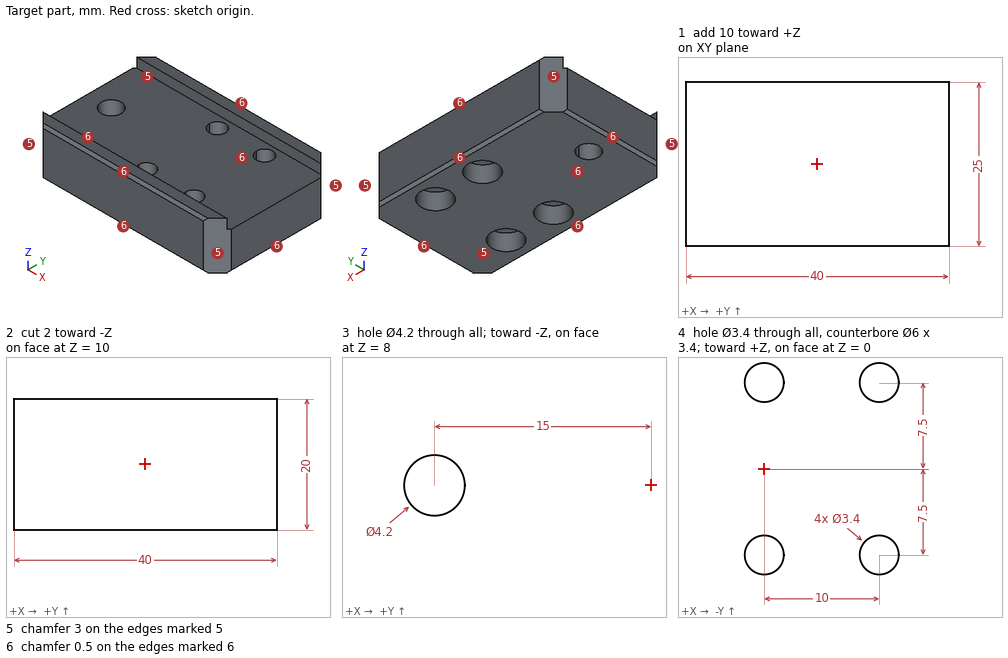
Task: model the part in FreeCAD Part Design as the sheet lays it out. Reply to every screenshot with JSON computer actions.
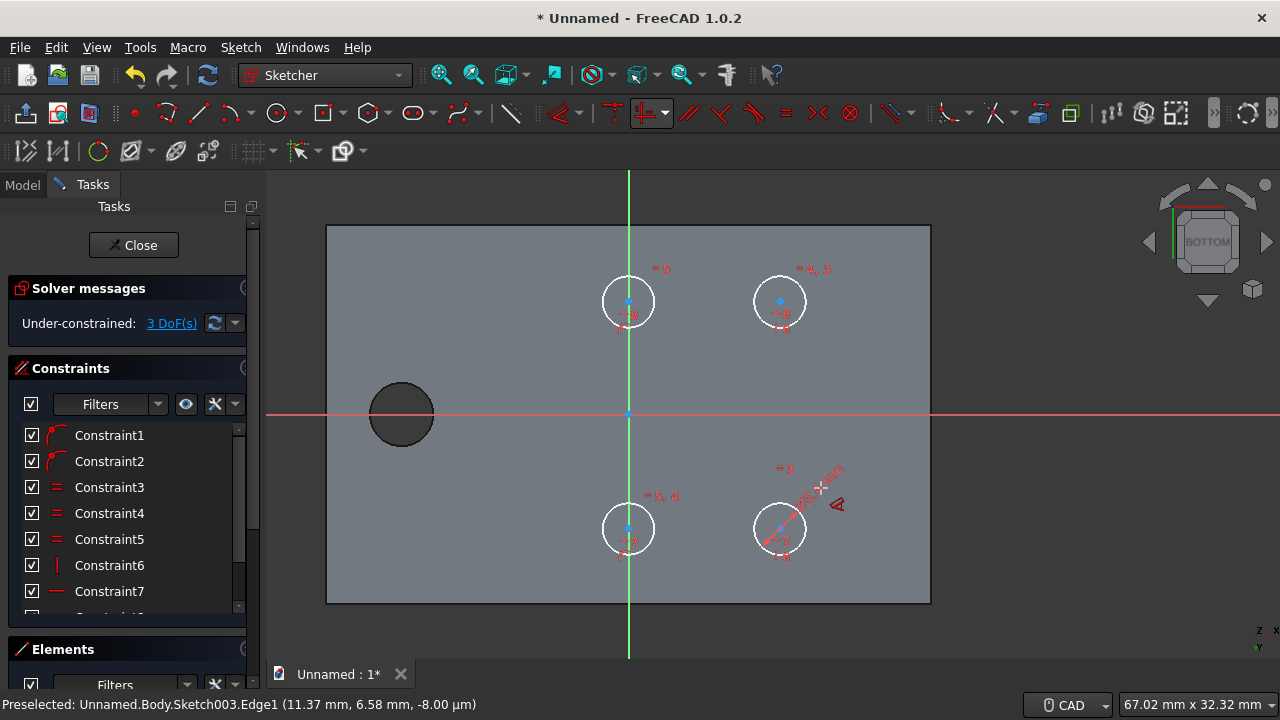
{"action": "left_click", "coordinate": [780, 529]}
{"action": "left_click", "coordinate": [704, 563]}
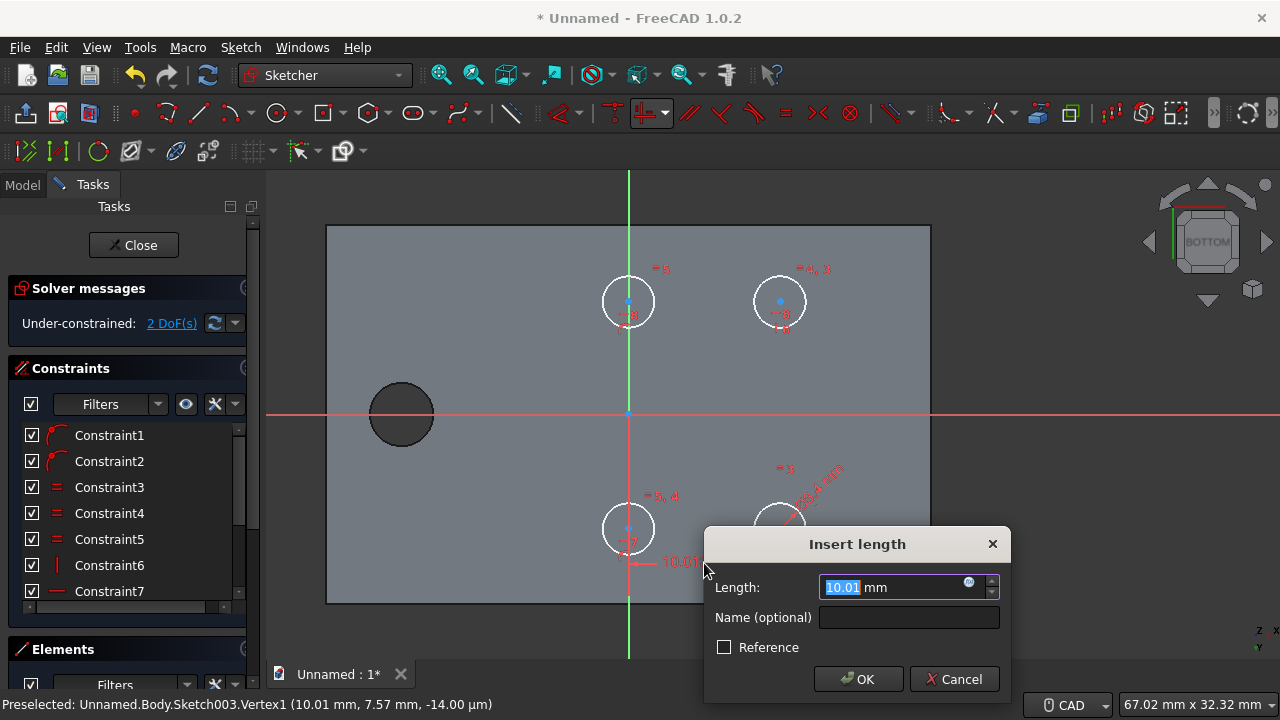
{"action": "type", "text": "10"}
{"action": "key", "text": "Return"}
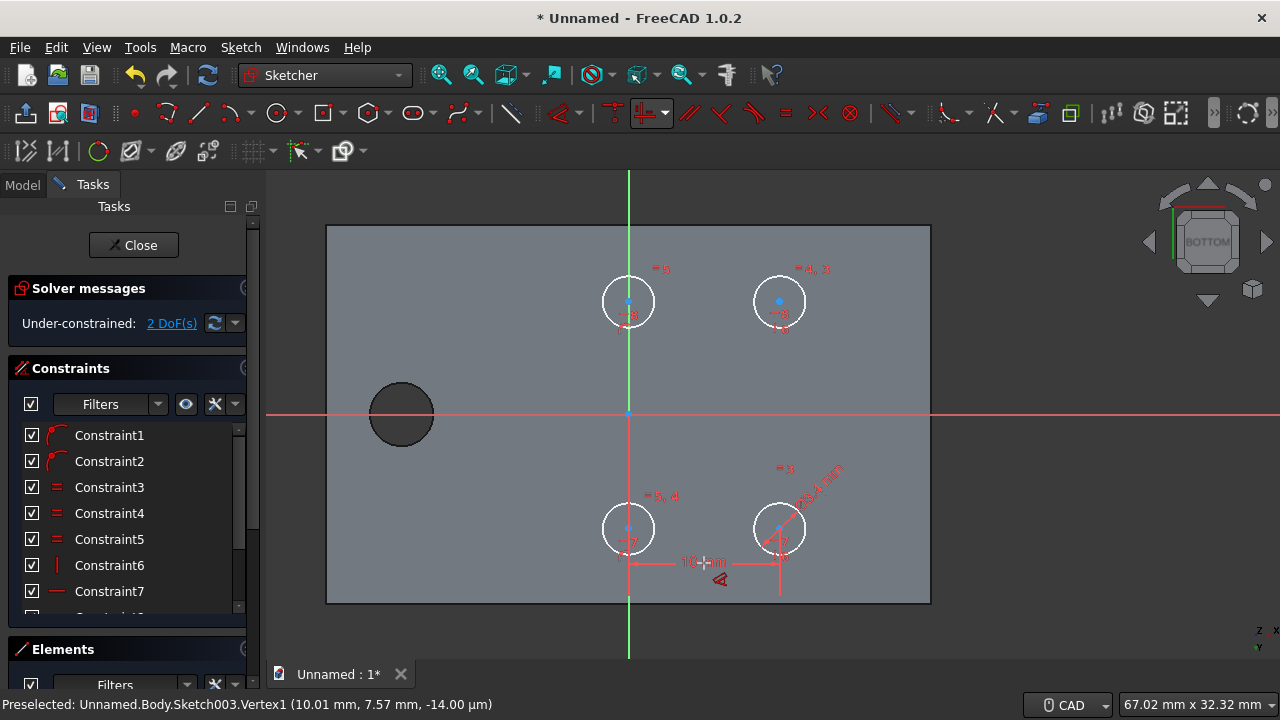
{"action": "left_click", "coordinate": [780, 529]}
{"action": "left_click", "coordinate": [814, 445]}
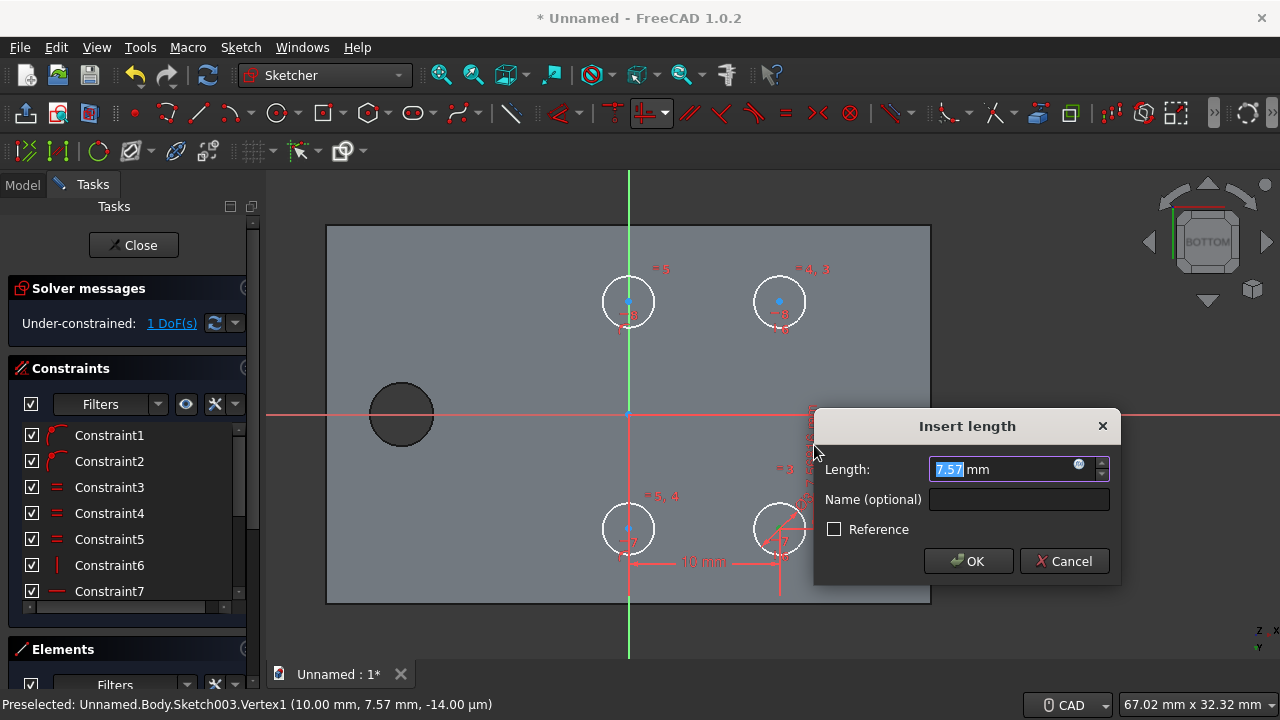
{"action": "type", "text": "7.5"}
{"action": "key", "text": "Return"}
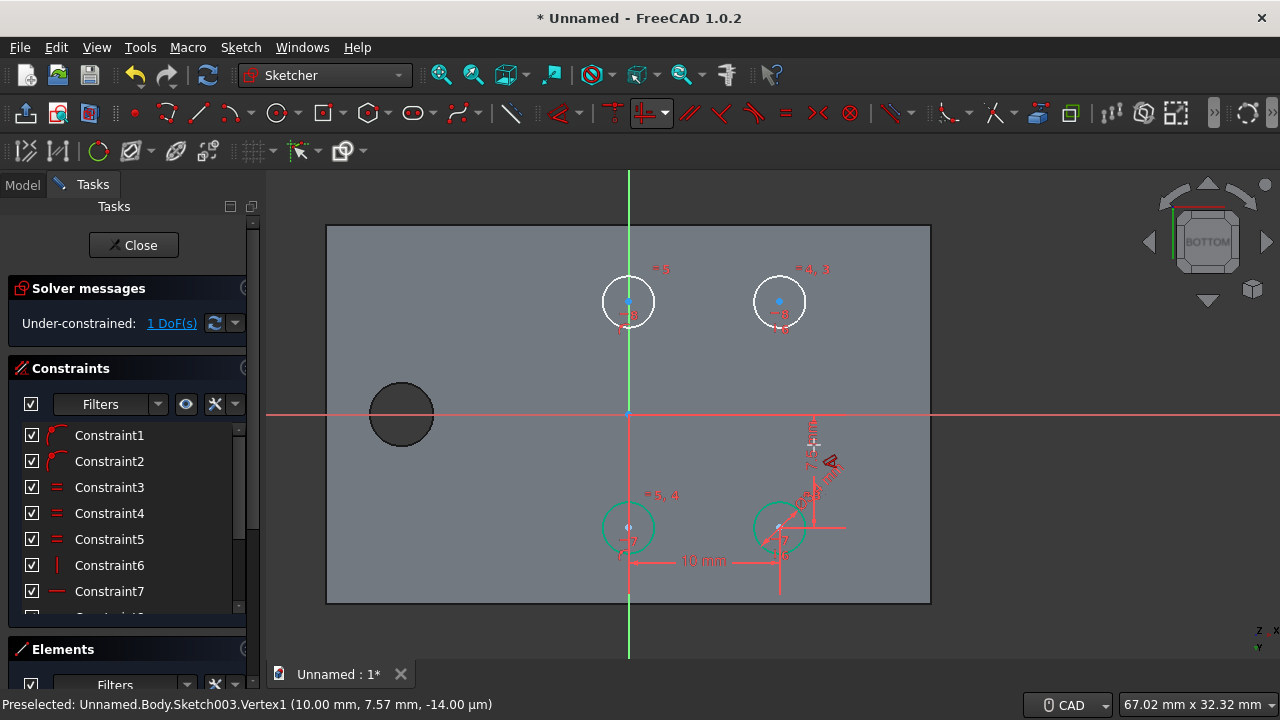
{"action": "left_click", "coordinate": [780, 302]}
{"action": "left_click", "coordinate": [814, 358]}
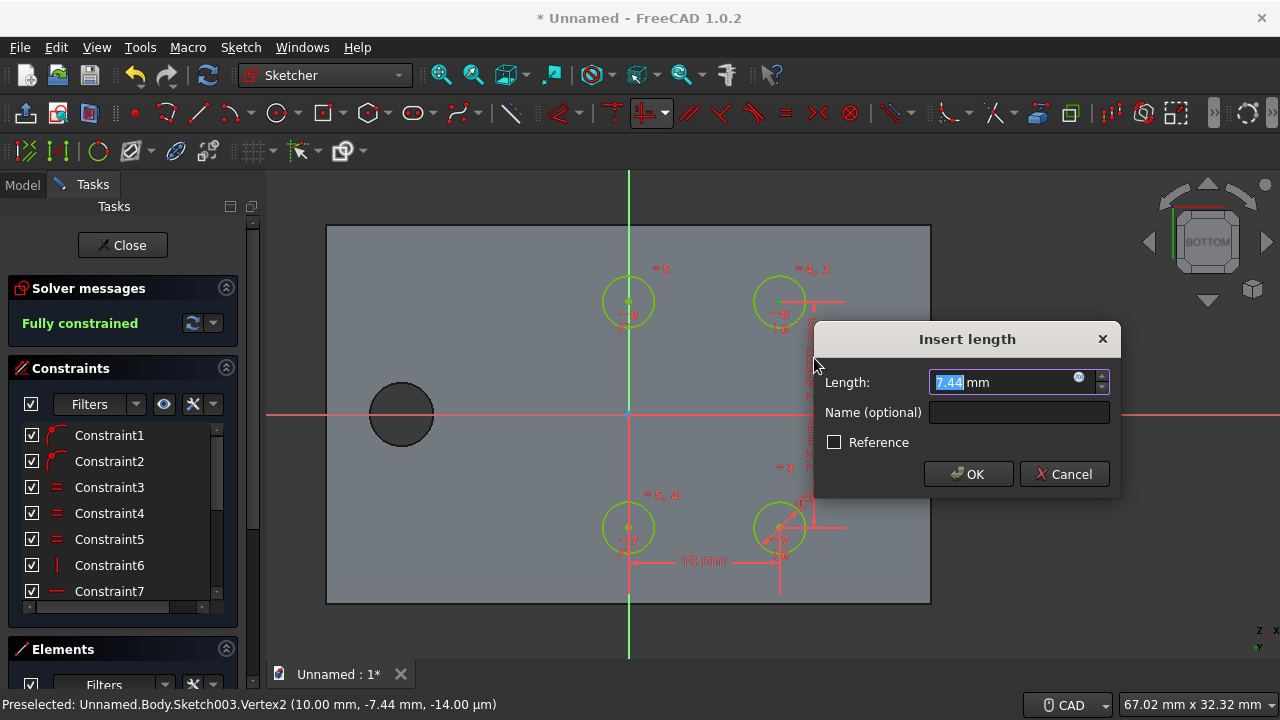
{"action": "type", "text": "7.5"}
{"action": "key", "text": "Return"}
{"action": "key", "text": "Escape"}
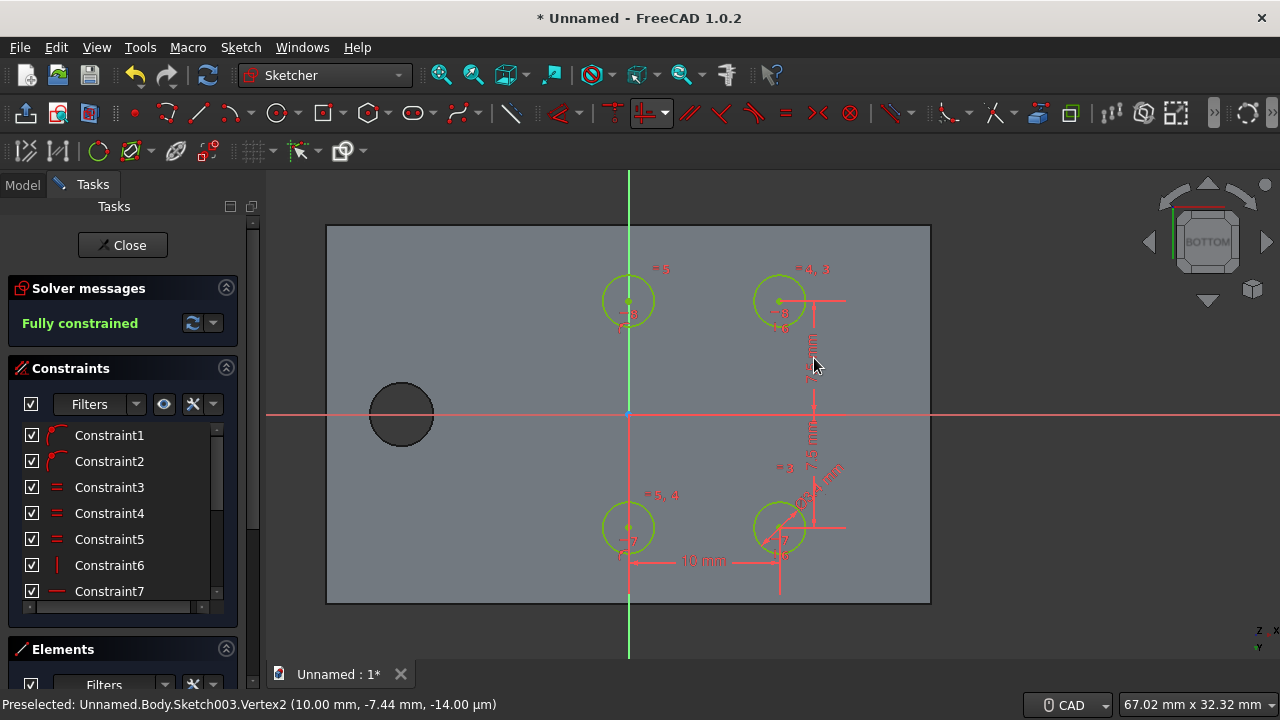
{"action": "left_click", "coordinate": [123, 245]}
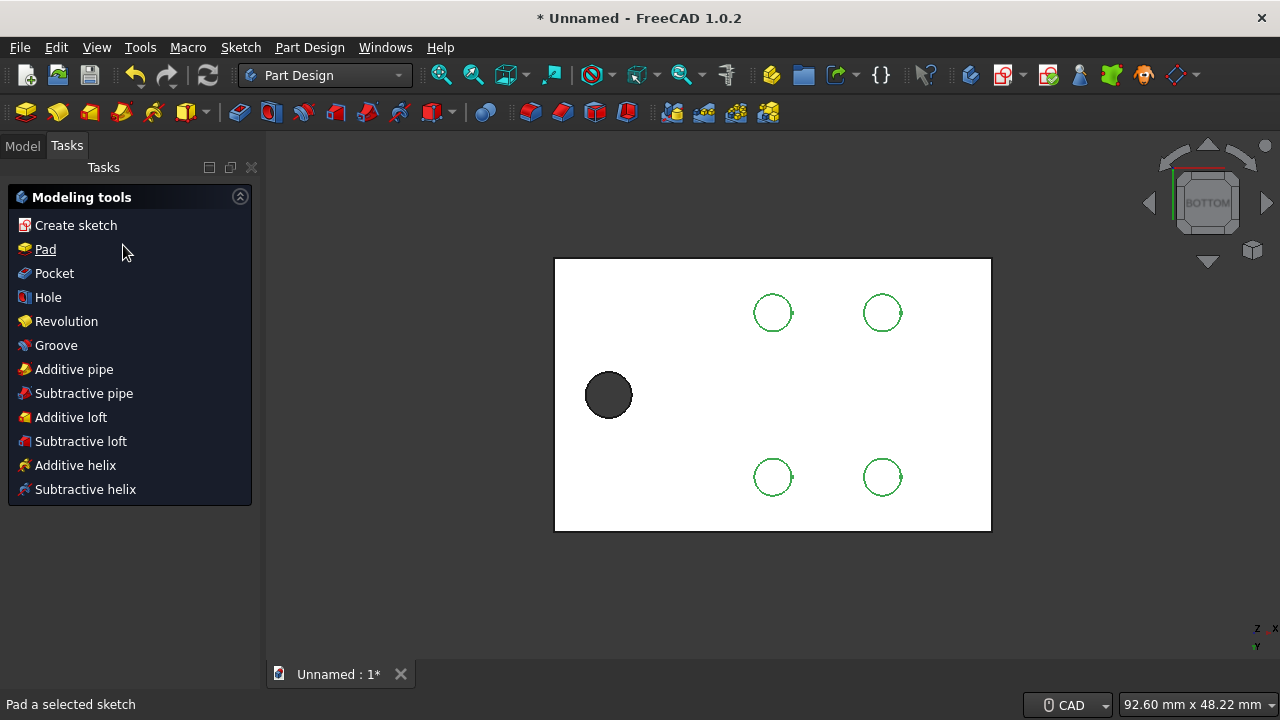
{"action": "left_click", "coordinate": [272, 112]}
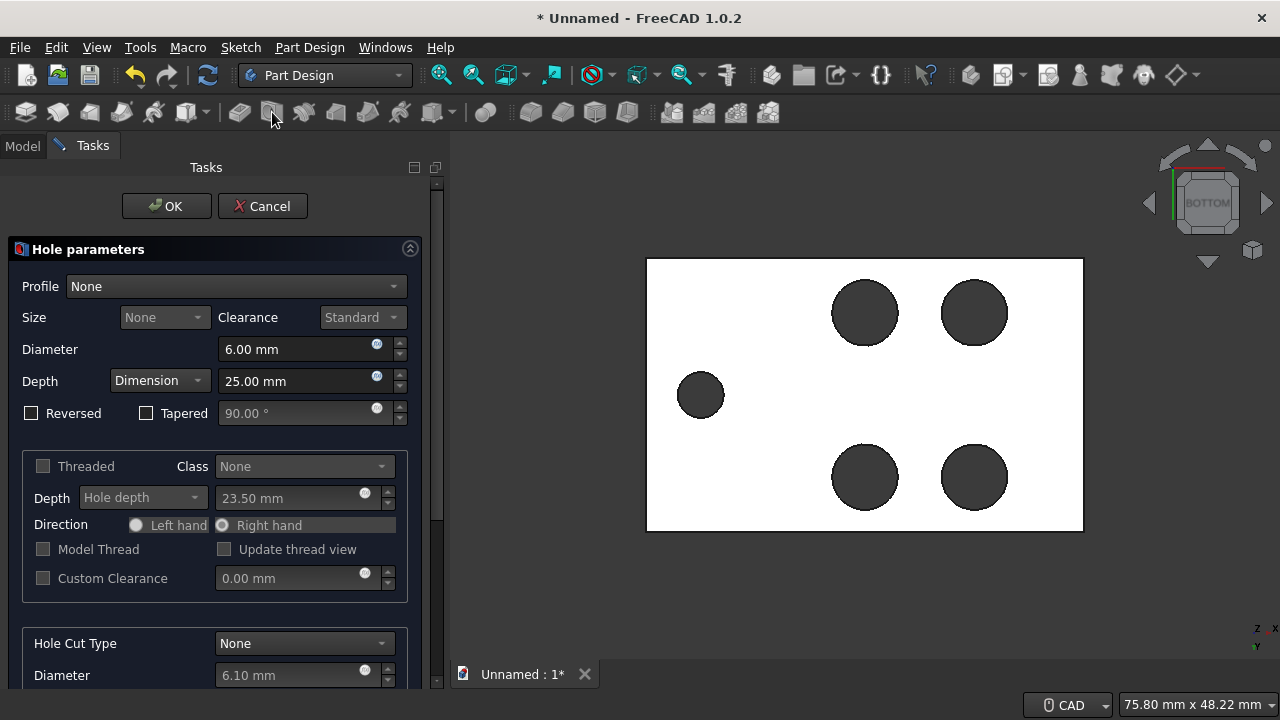
{"action": "triple_click", "coordinate": [305, 349]}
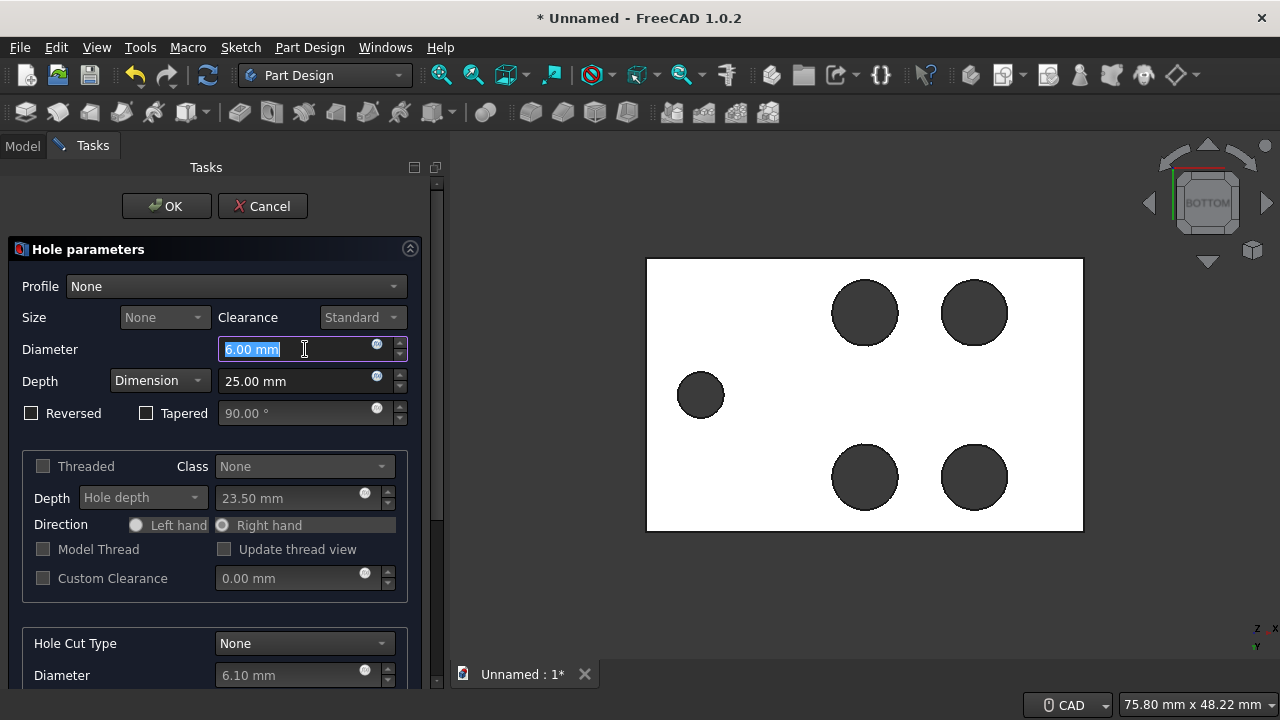
{"action": "type", "text": "3.4"}
{"action": "key", "text": "Tab"}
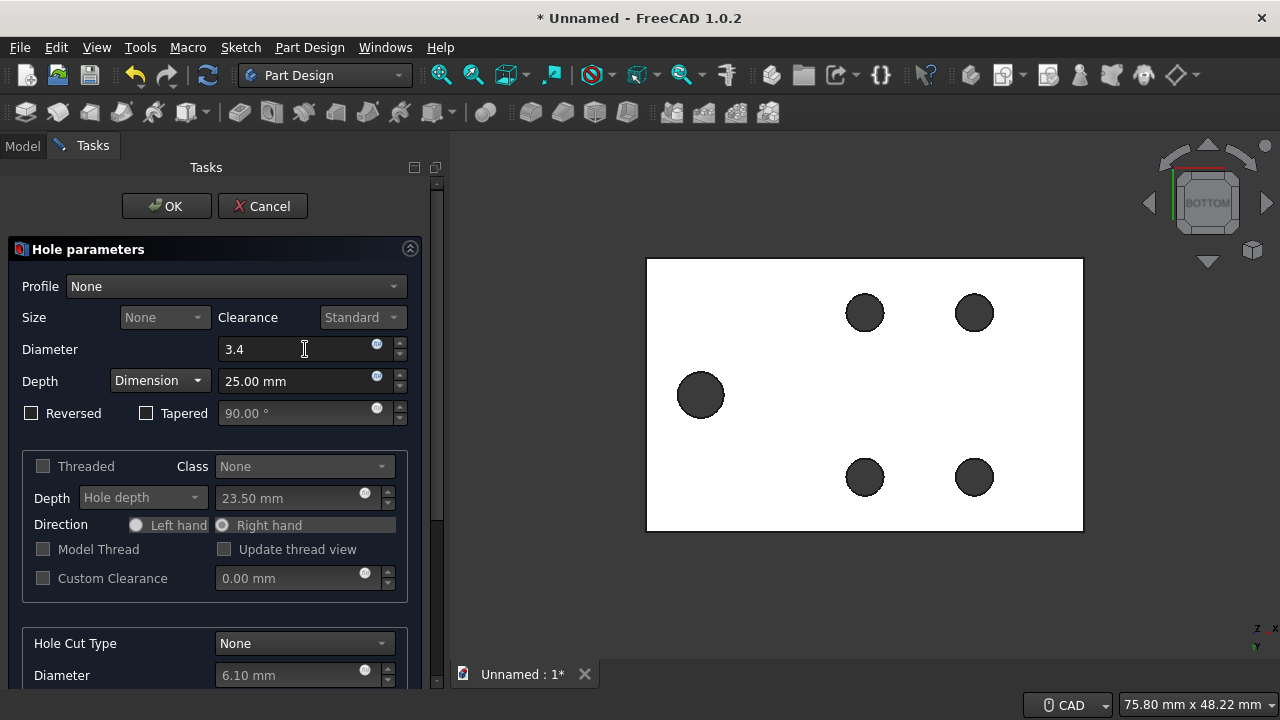
{"action": "left_click", "coordinate": [161, 380]}